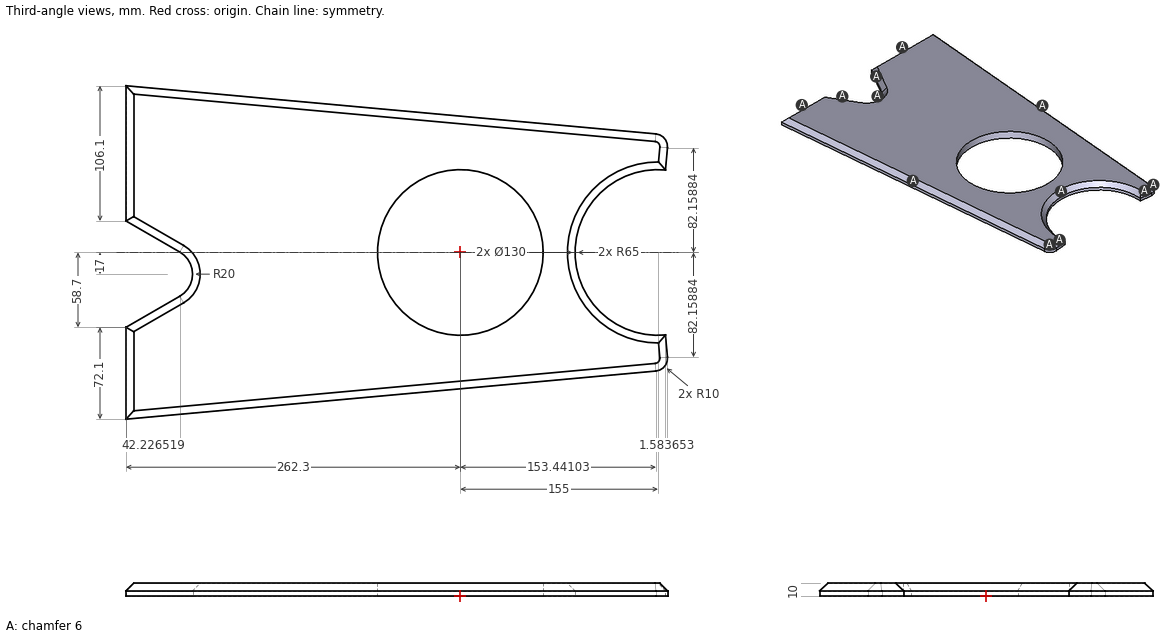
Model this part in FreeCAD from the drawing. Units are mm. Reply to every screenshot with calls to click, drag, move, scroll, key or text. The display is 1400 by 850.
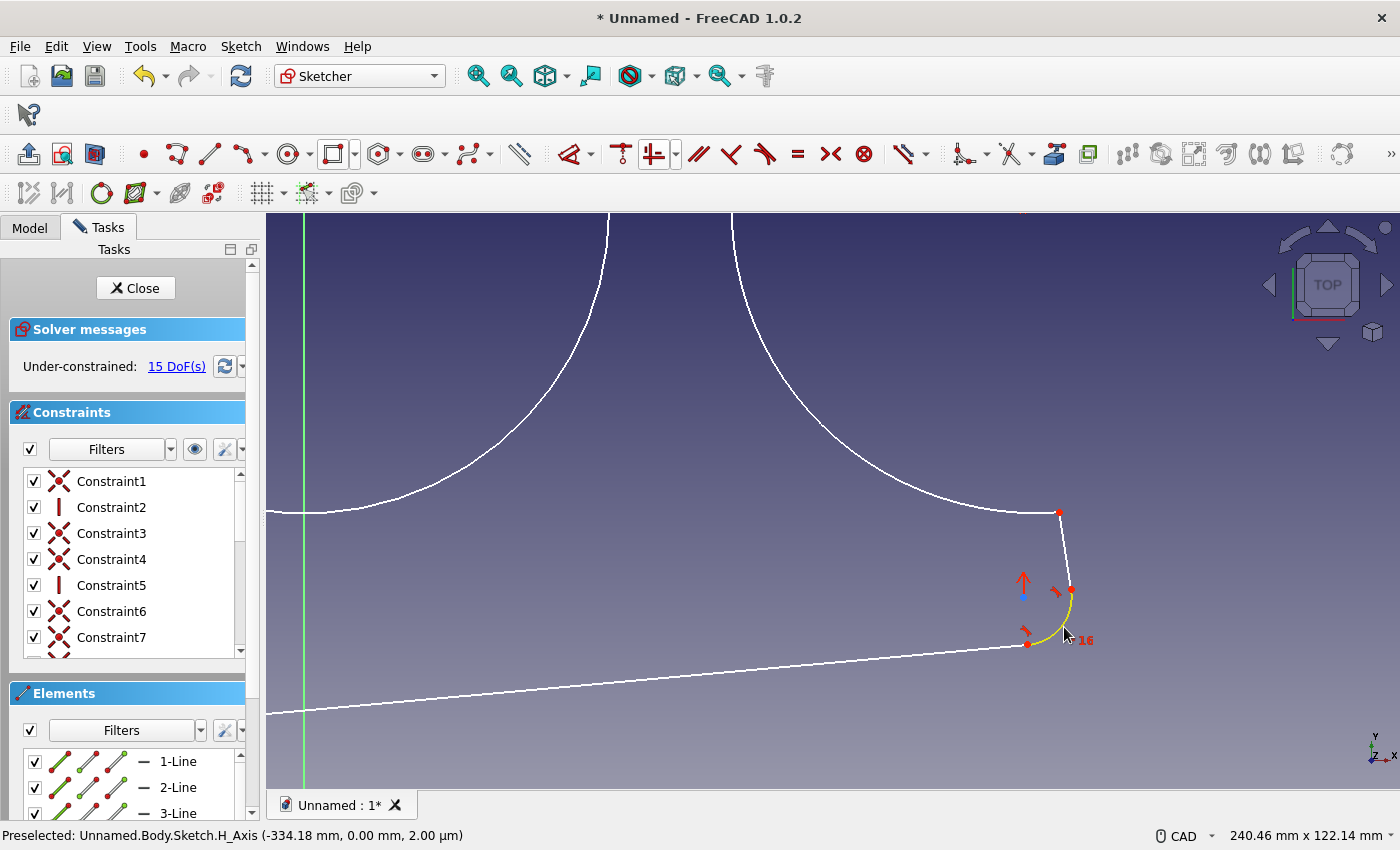
click(1061, 627)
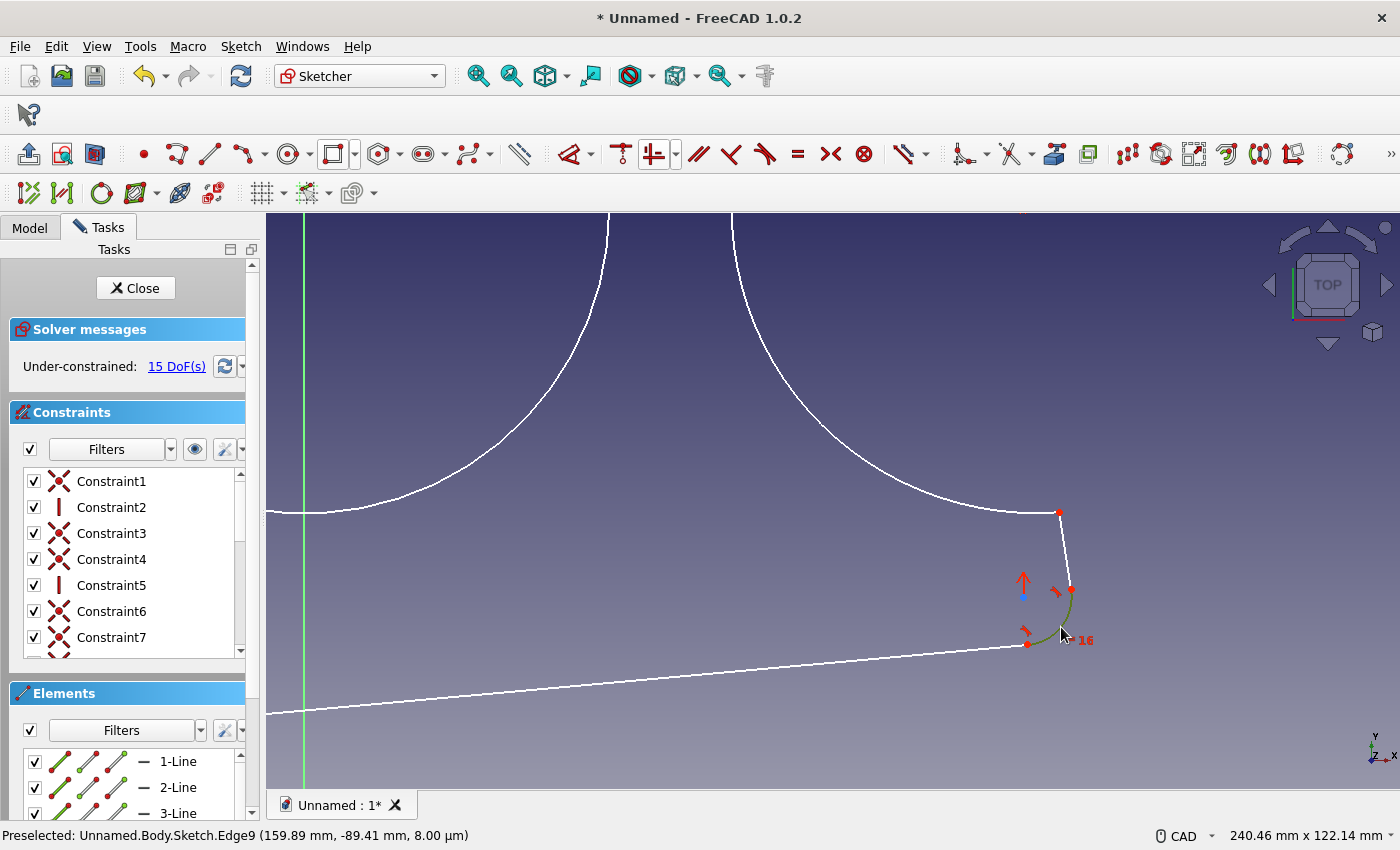
key(k)
key(r)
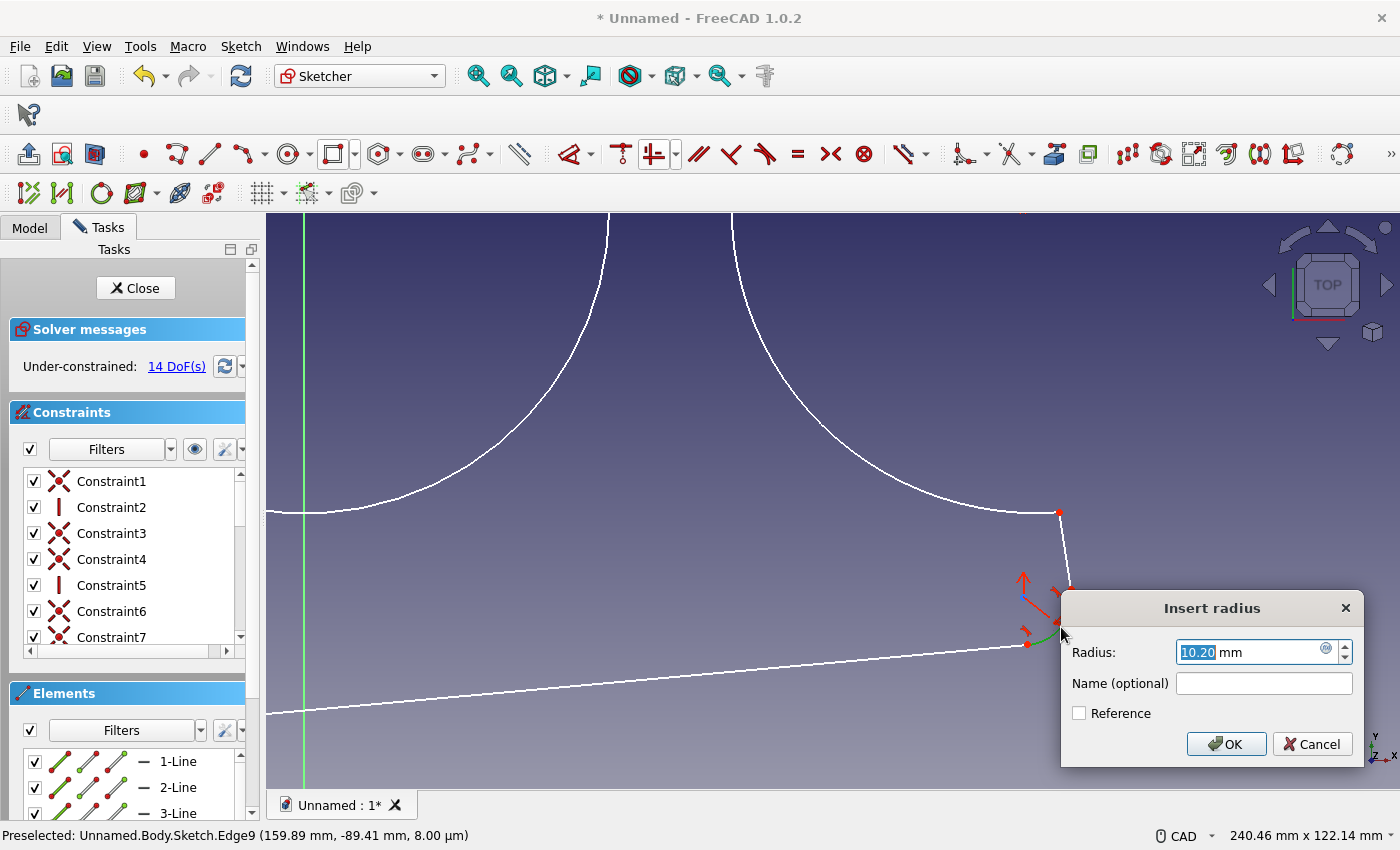
text(10)
key(Return)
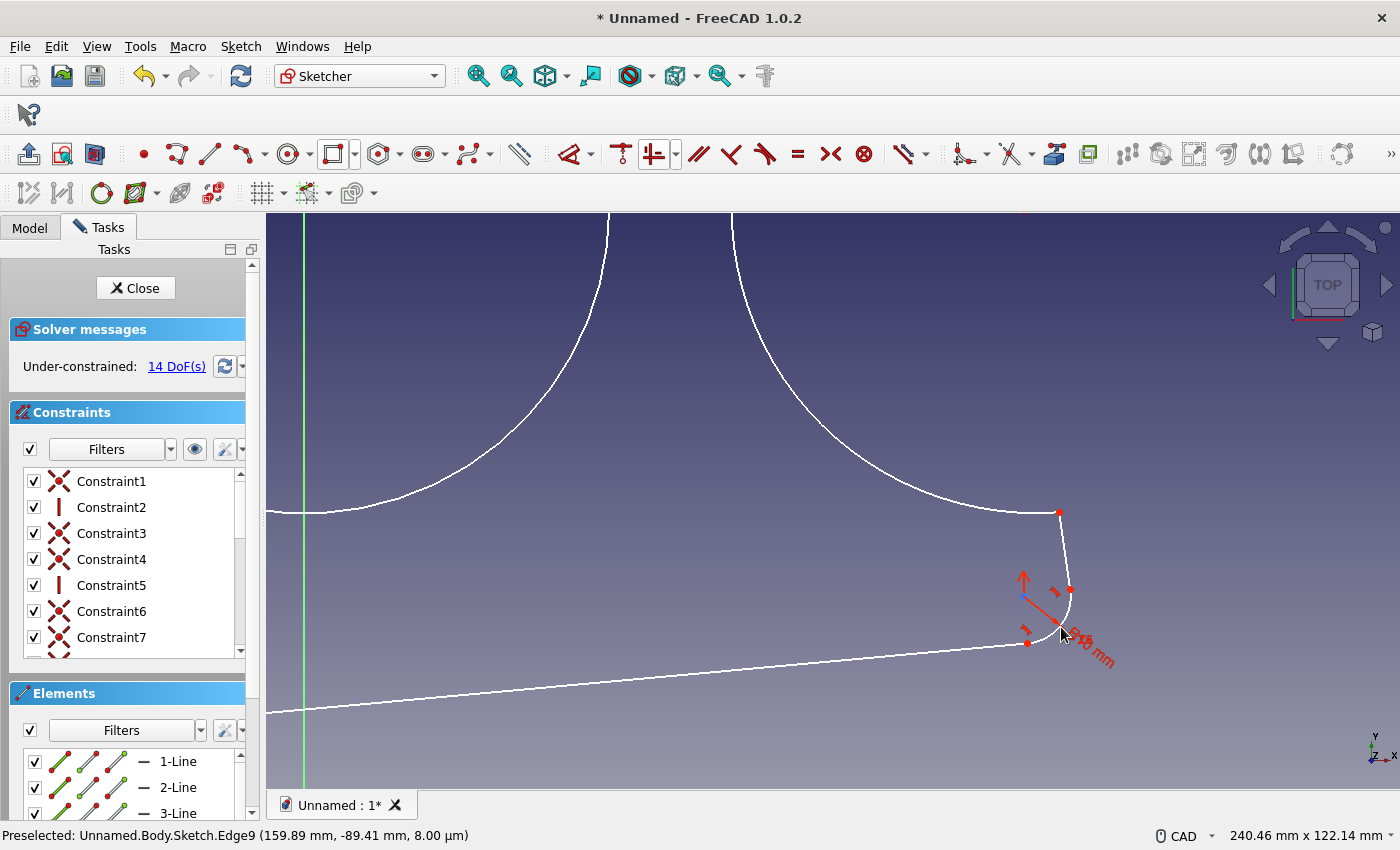
click(795, 394)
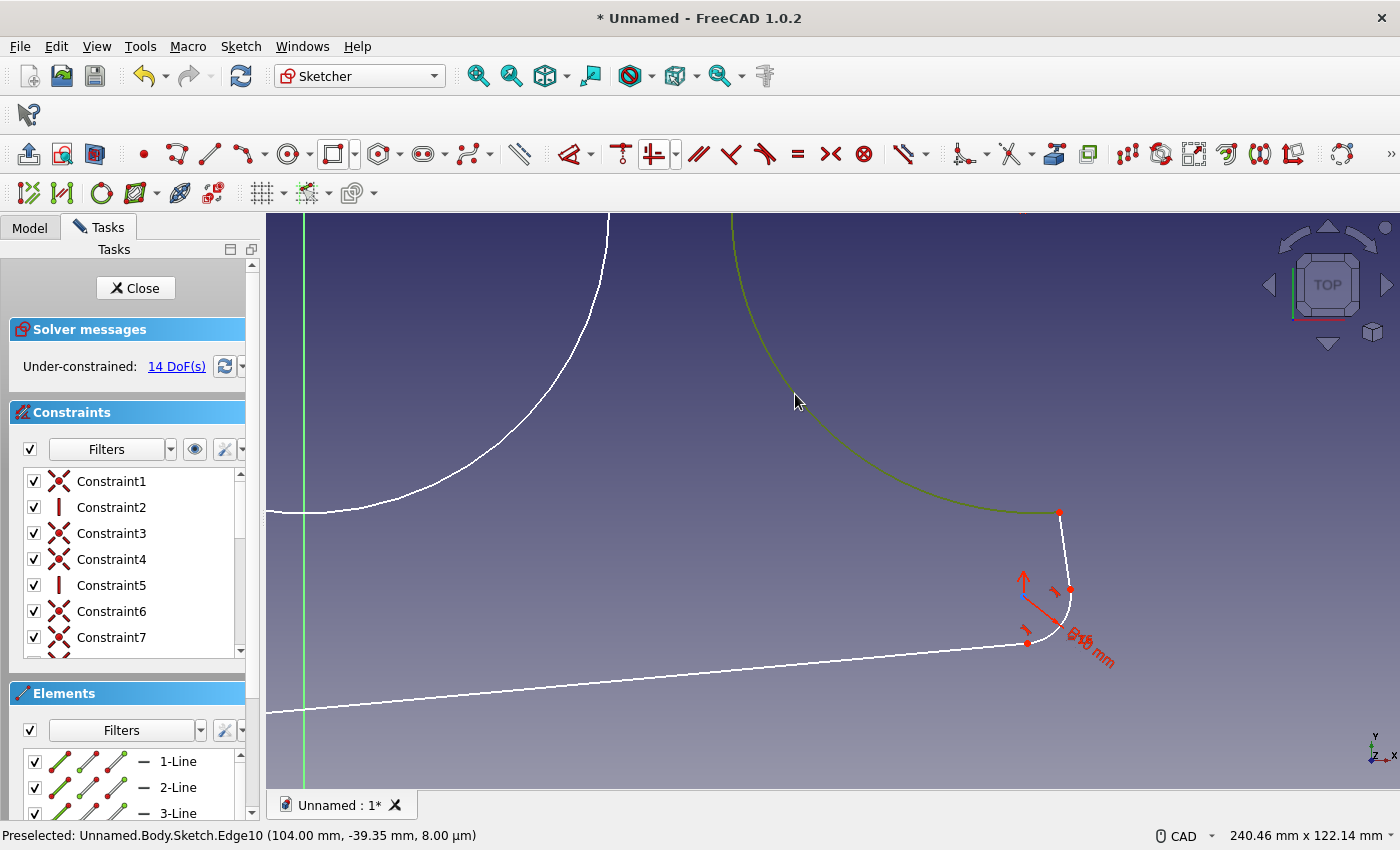
click(590, 154)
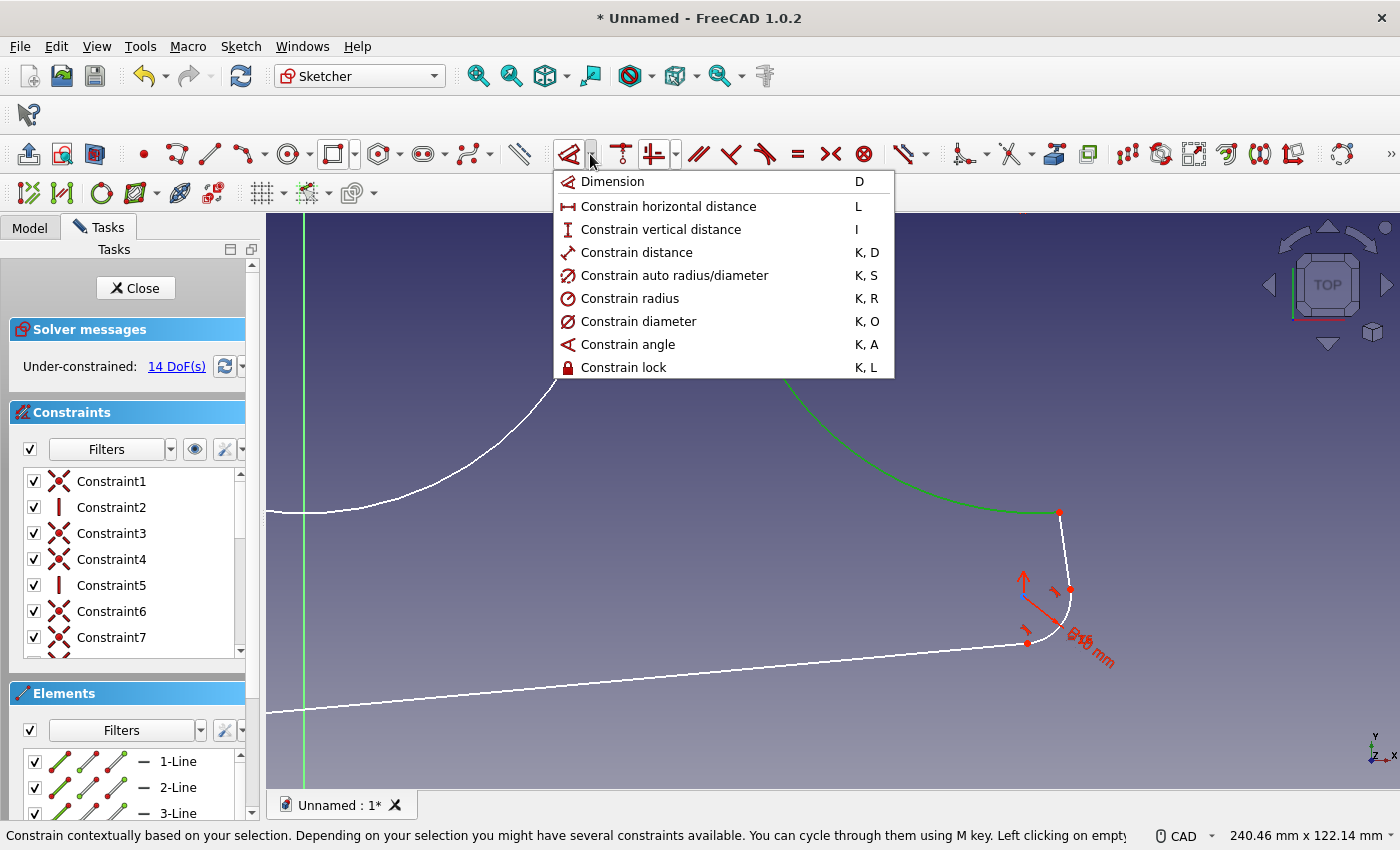
click(724, 298)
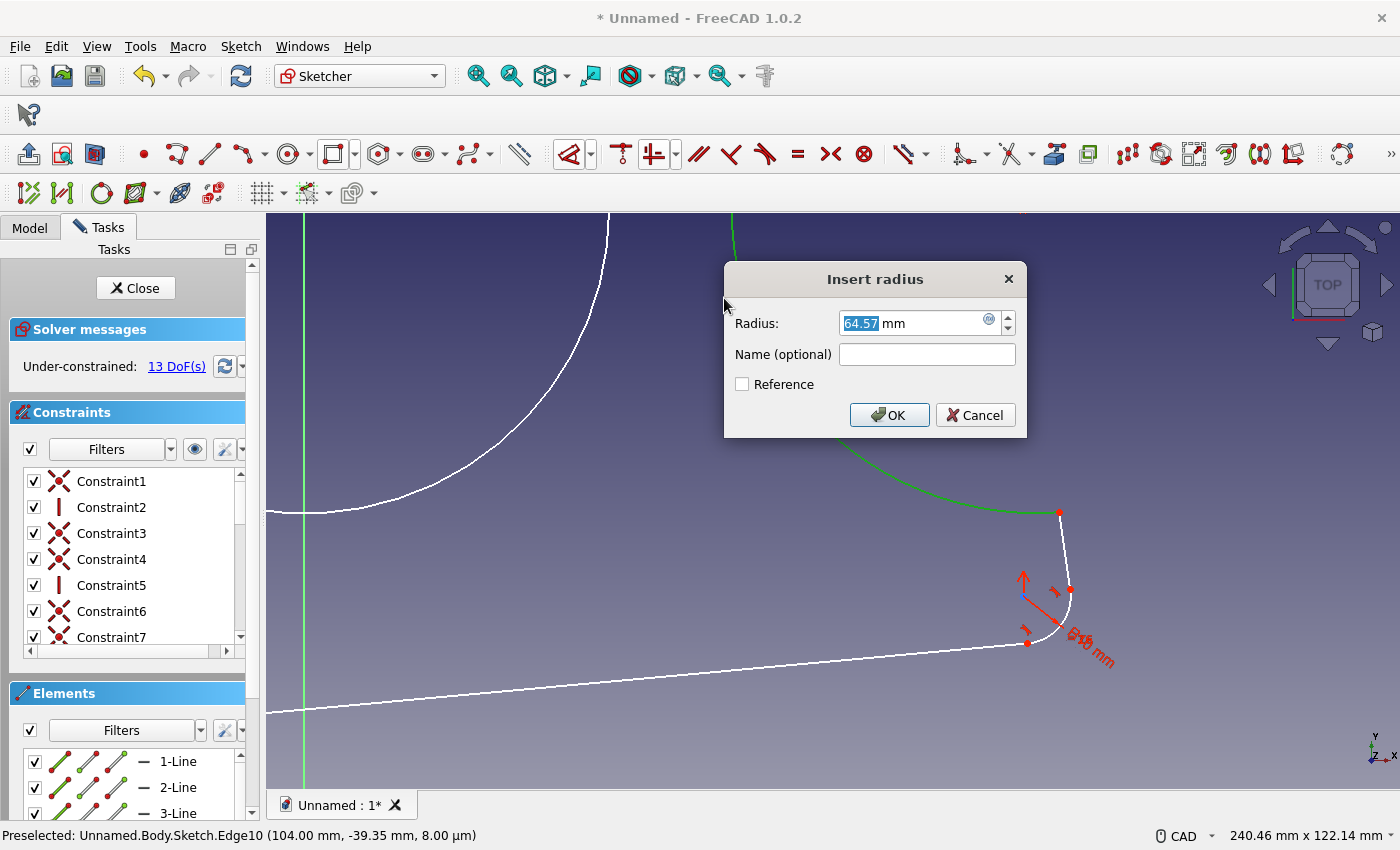
text(65)
key(Return)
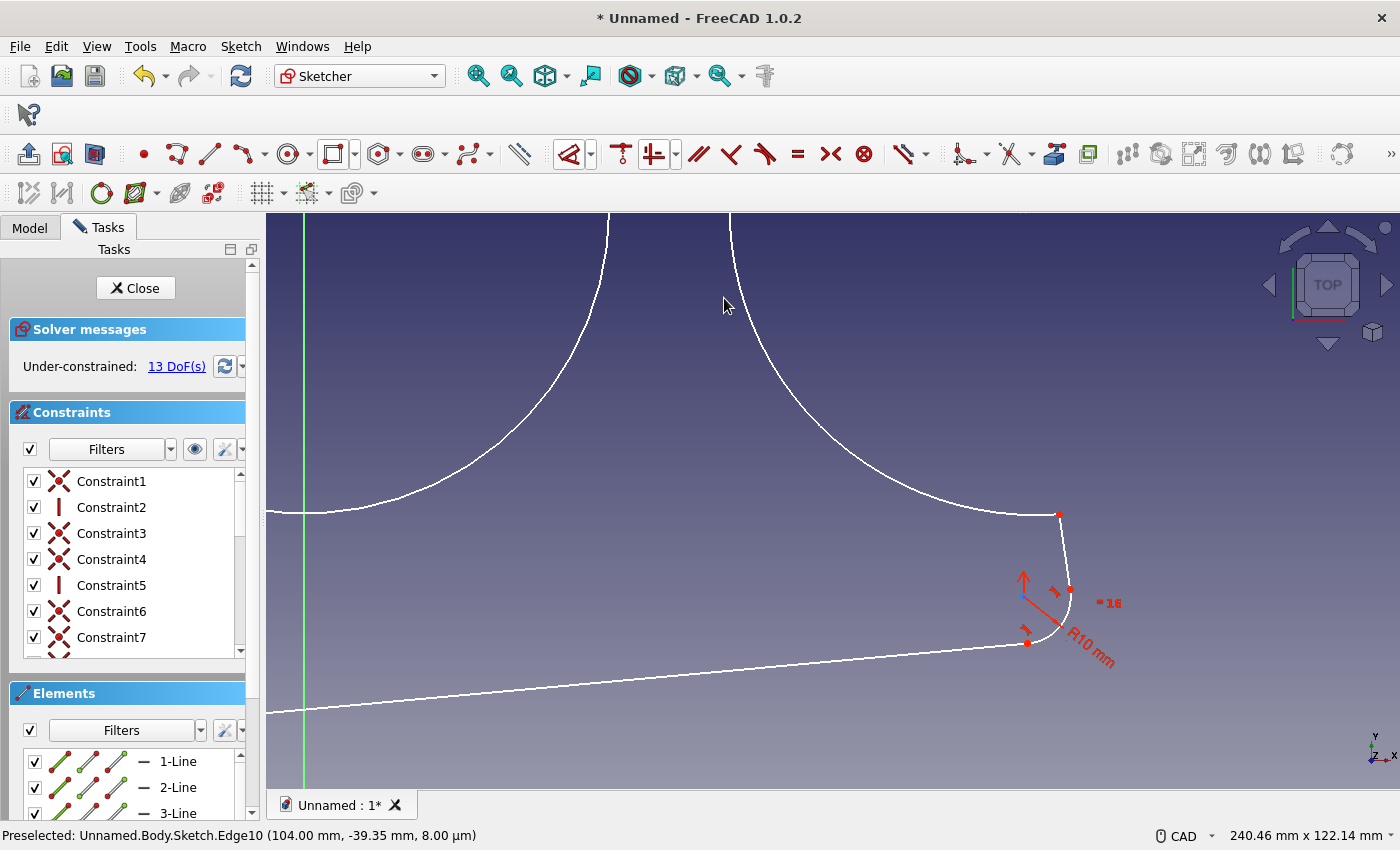
scroll(1064, 627, down, 6)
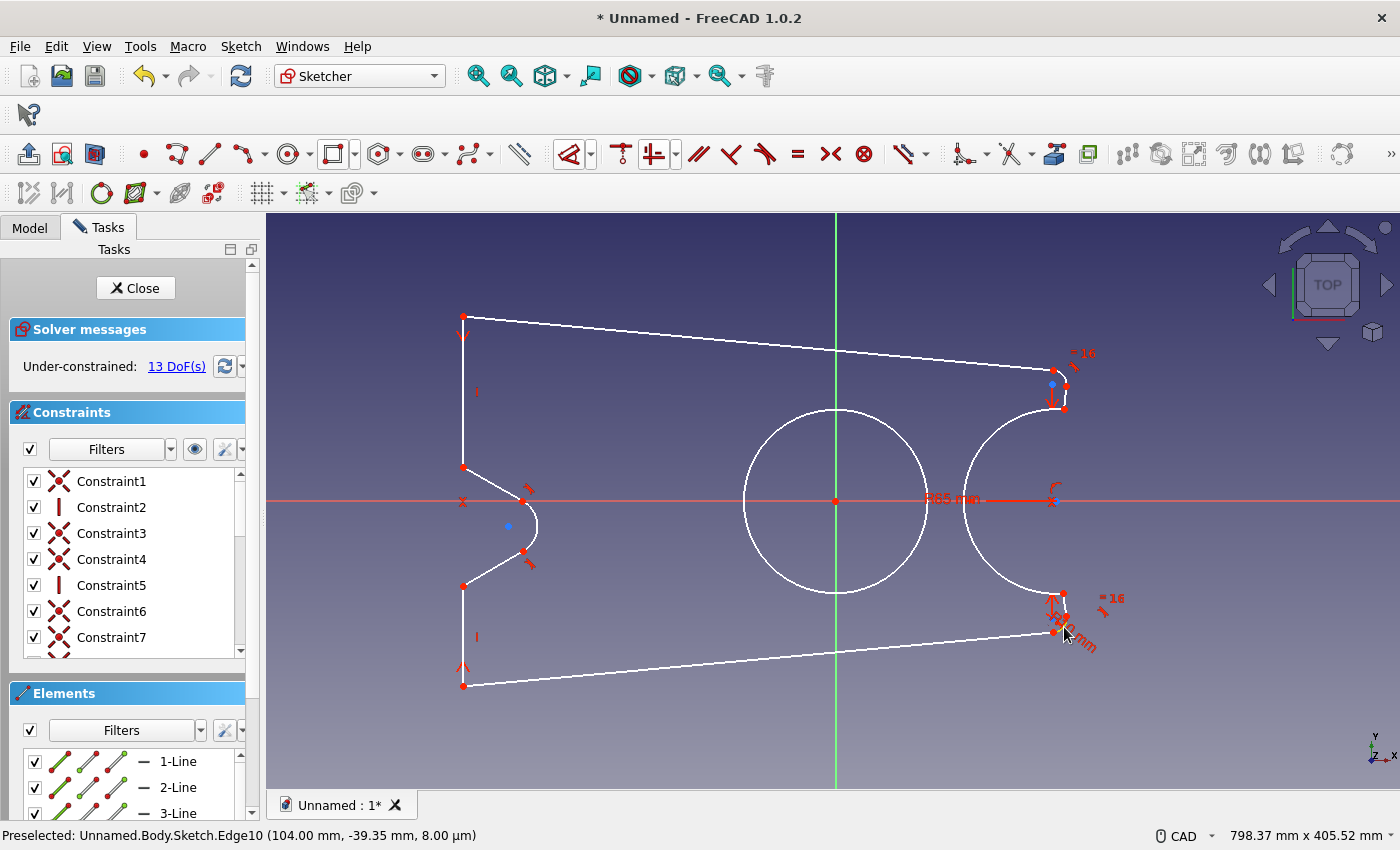
scroll(535, 538, up, 2)